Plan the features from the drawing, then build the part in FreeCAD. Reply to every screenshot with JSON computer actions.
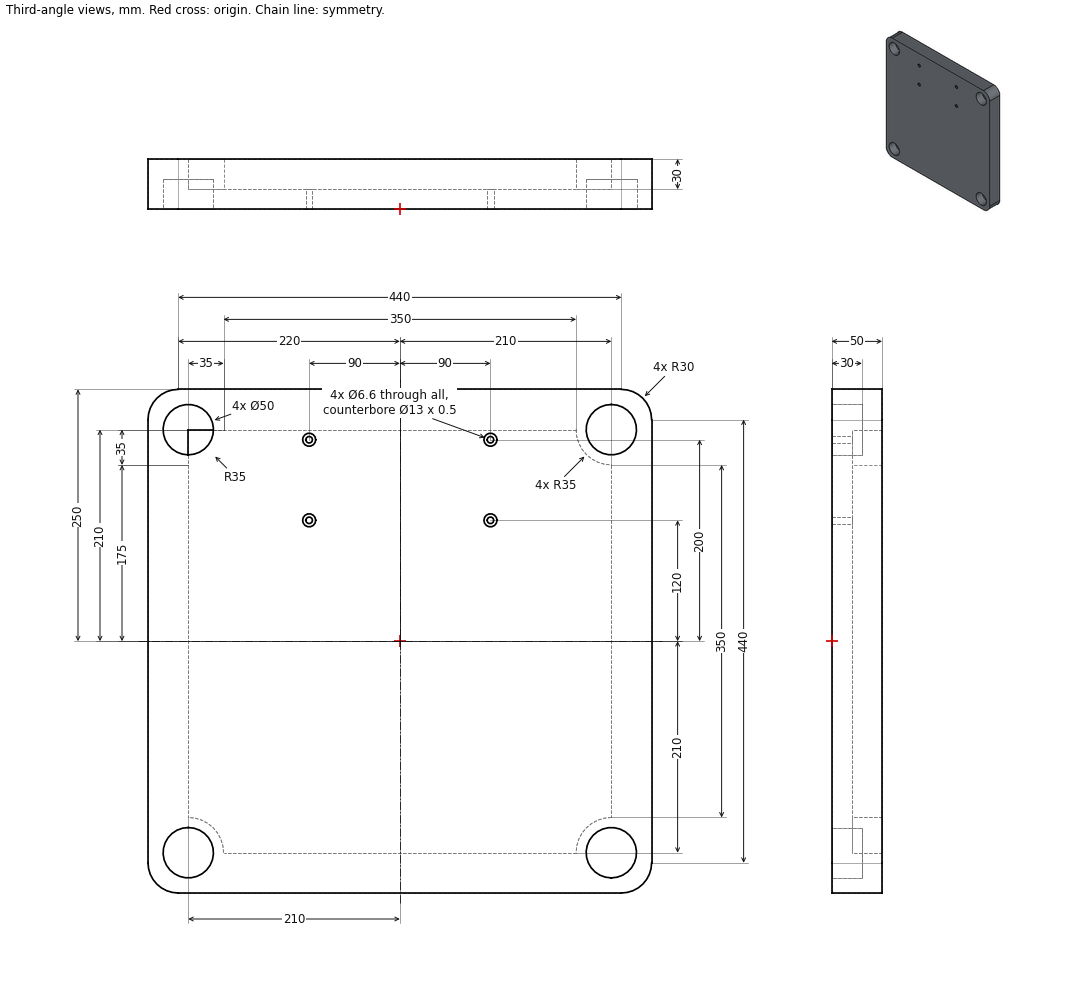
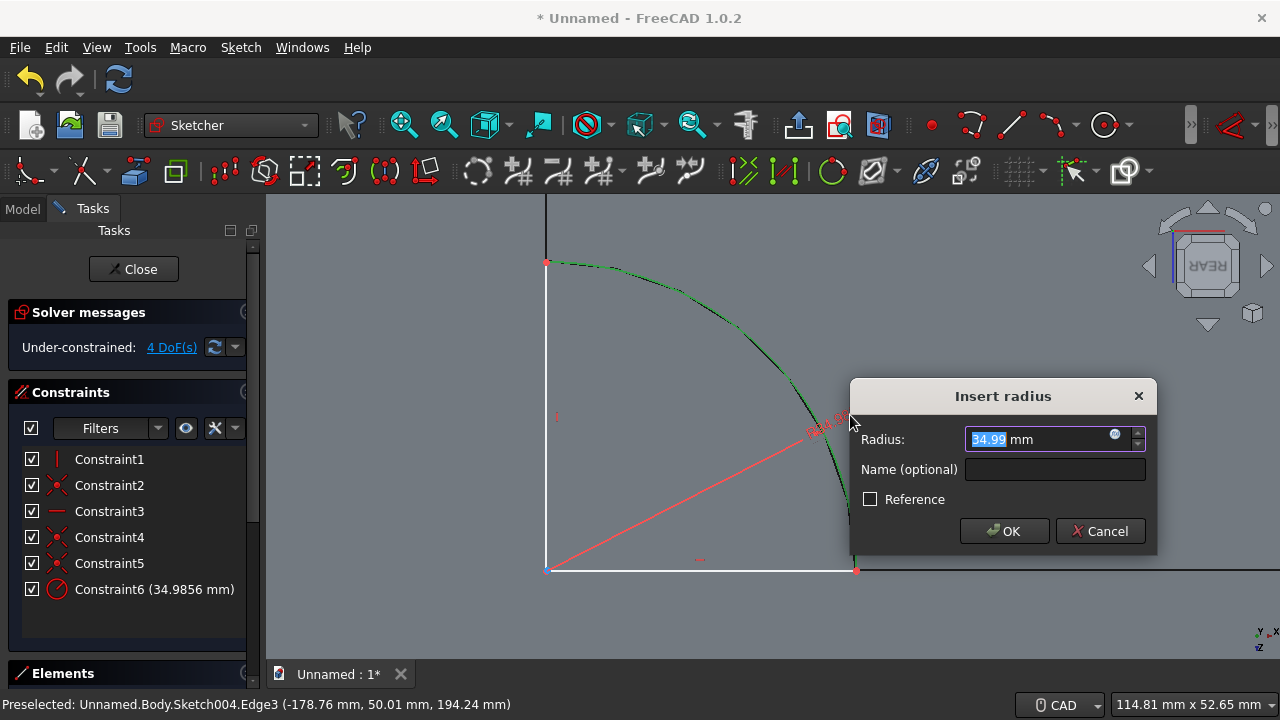
{"action": "type", "text": "35"}
{"action": "key", "text": "Return"}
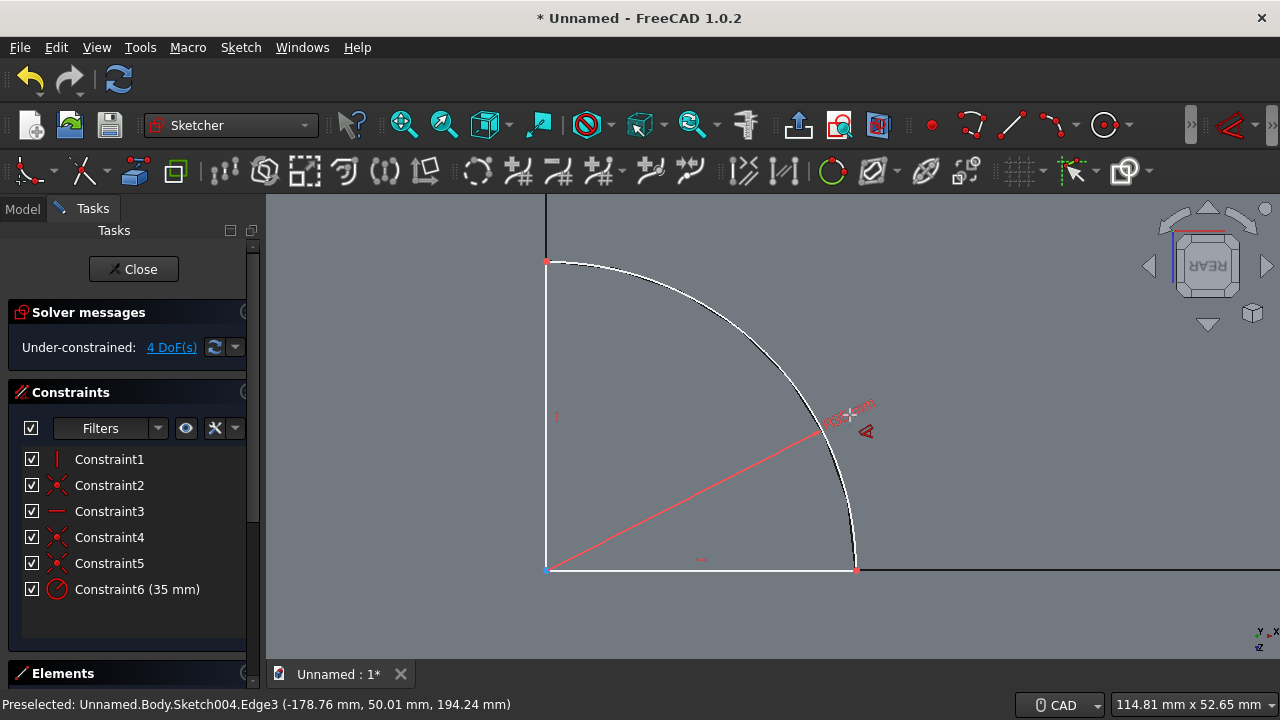
{"action": "left_click", "coordinate": [546, 355]}
{"action": "left_click", "coordinate": [512, 416]}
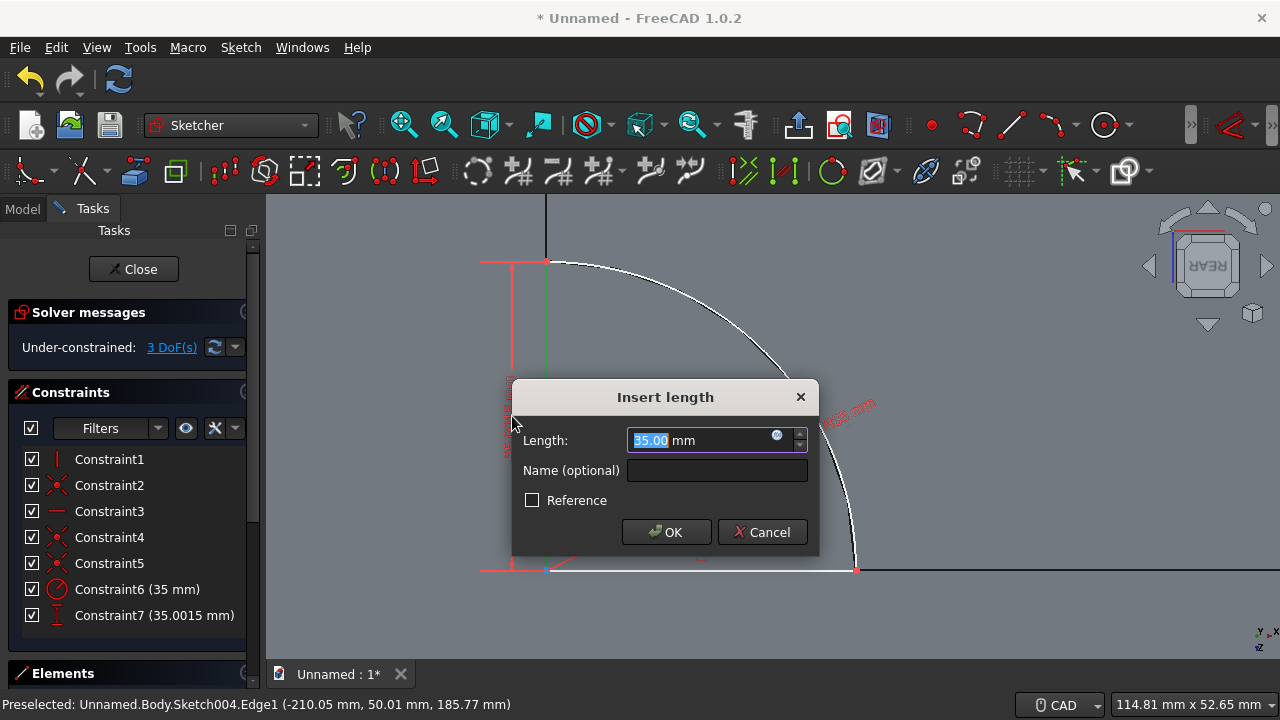
{"action": "type", "text": "35"}
{"action": "key", "text": "Return"}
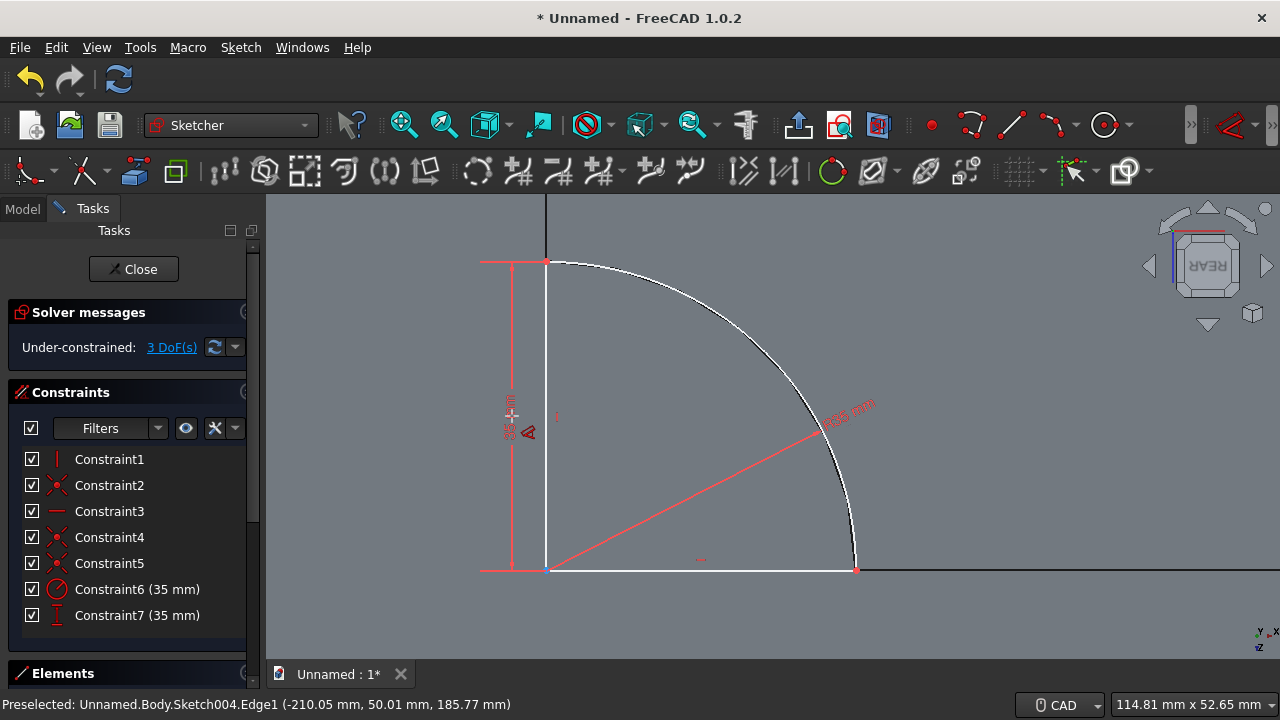
{"action": "left_click", "coordinate": [639, 571]}
{"action": "left_click", "coordinate": [701, 605]}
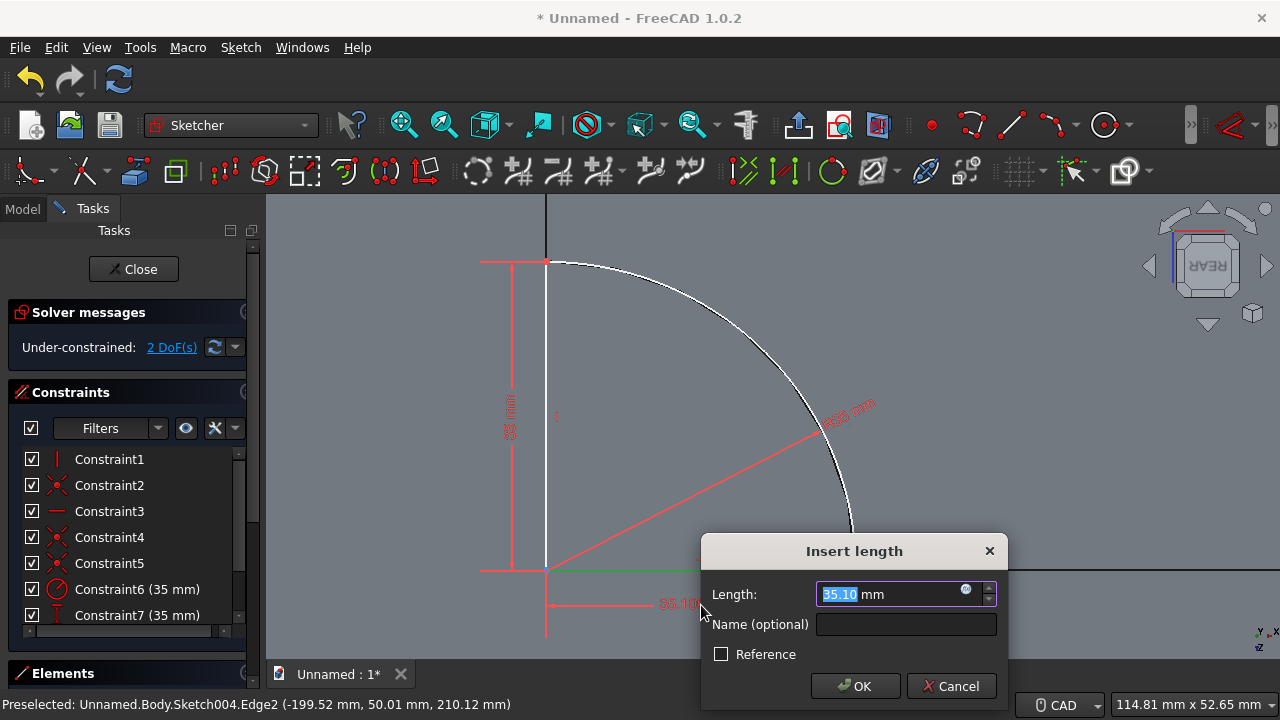
{"action": "type", "text": "35"}
{"action": "key", "text": "Return"}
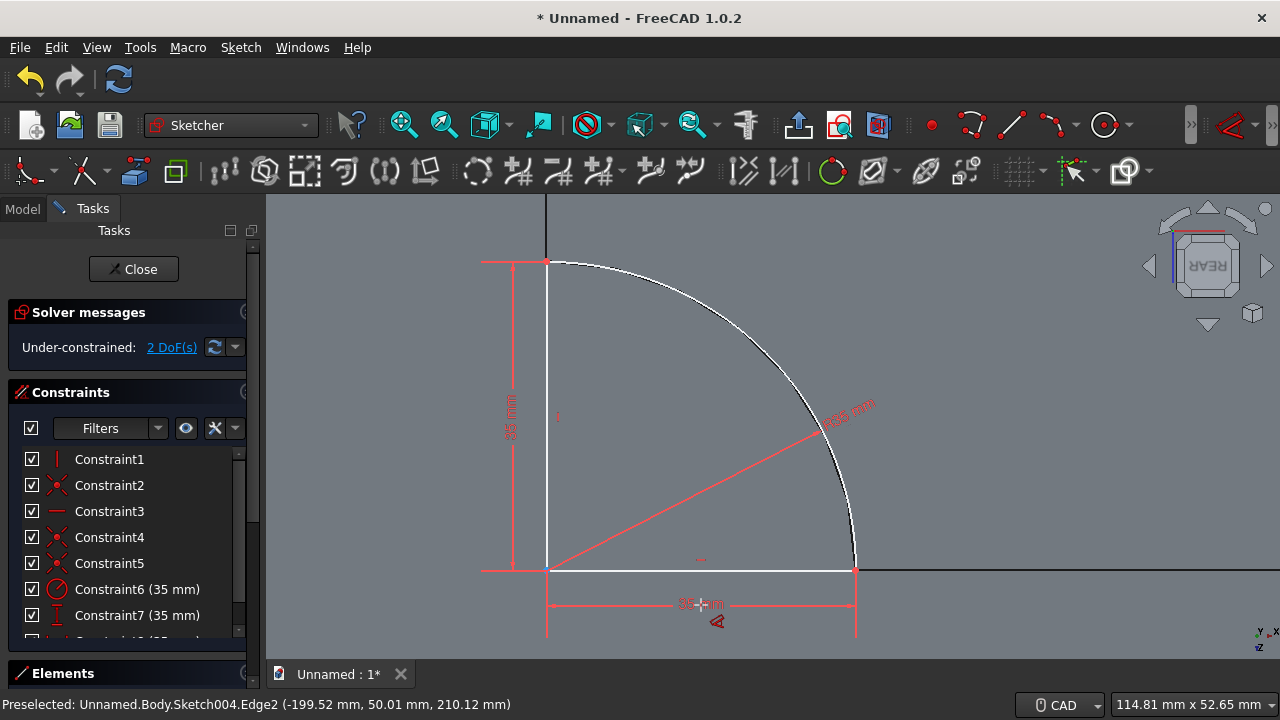
{"action": "left_click", "coordinate": [547, 262]}
{"action": "left_click", "coordinate": [831, 296]}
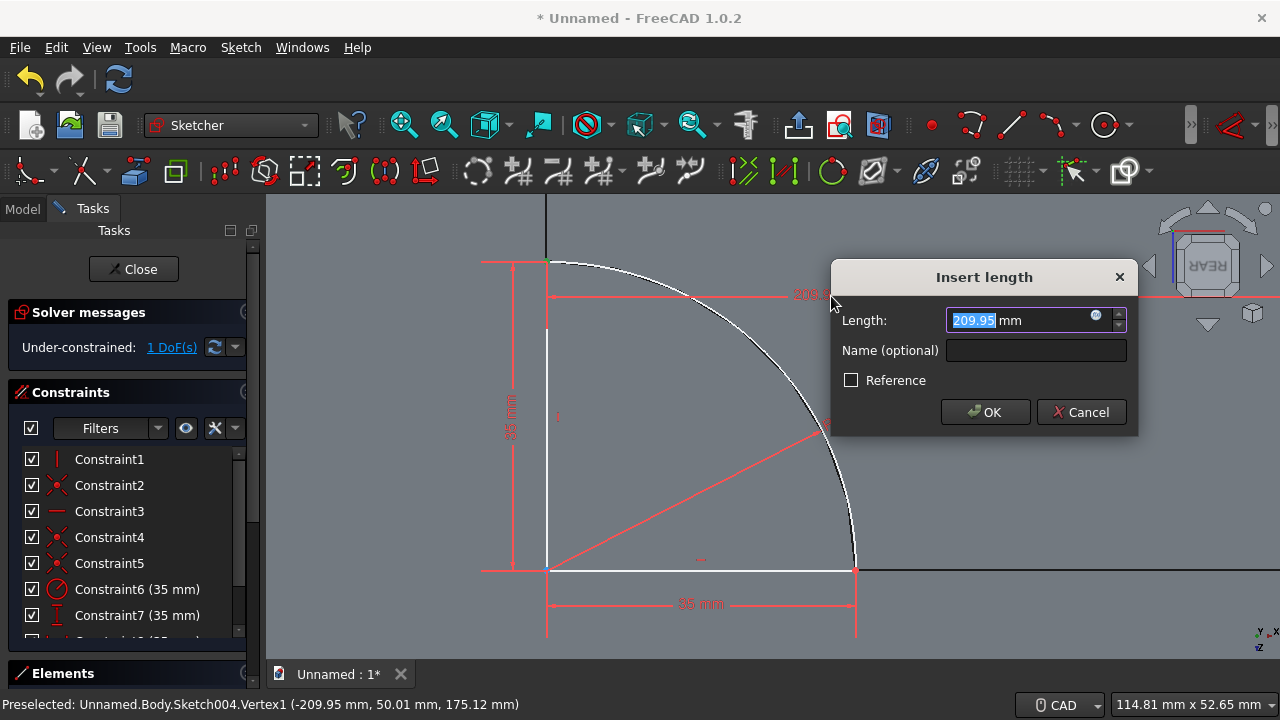
{"action": "type", "text": "210"}
{"action": "key", "text": "Return"}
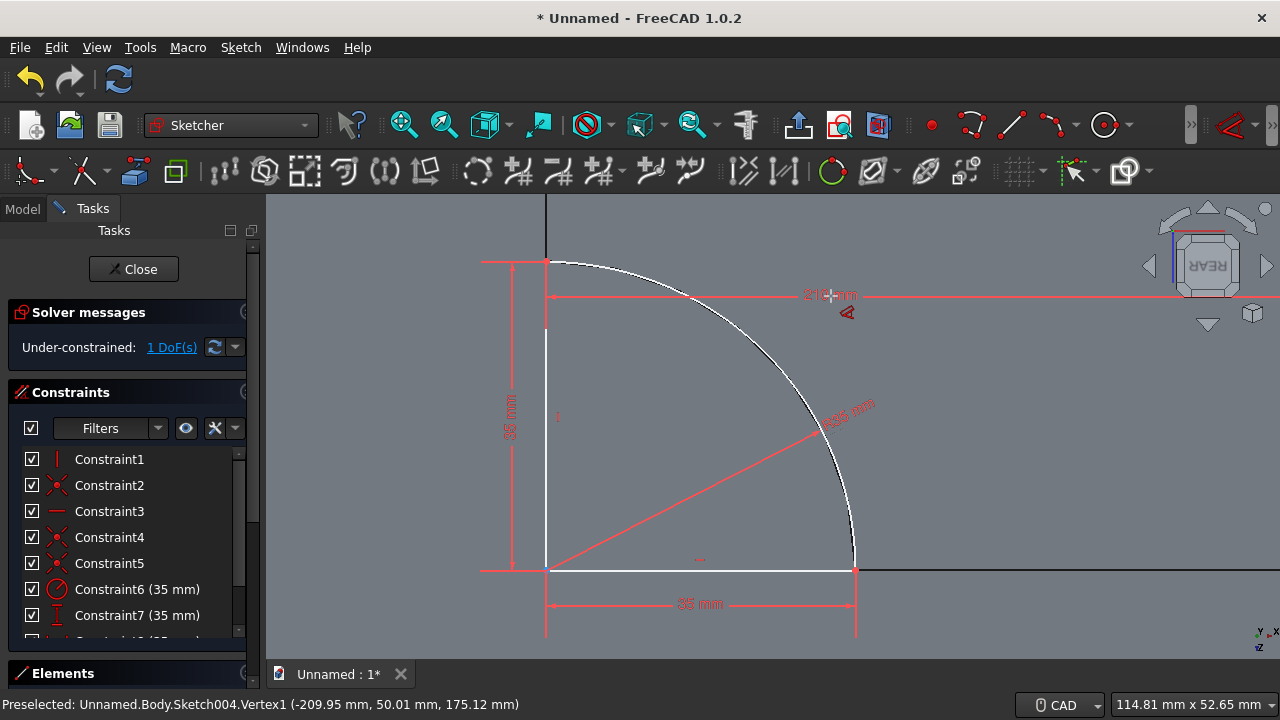
{"action": "left_click", "coordinate": [546, 262]}
{"action": "left_click", "coordinate": [512, 242]}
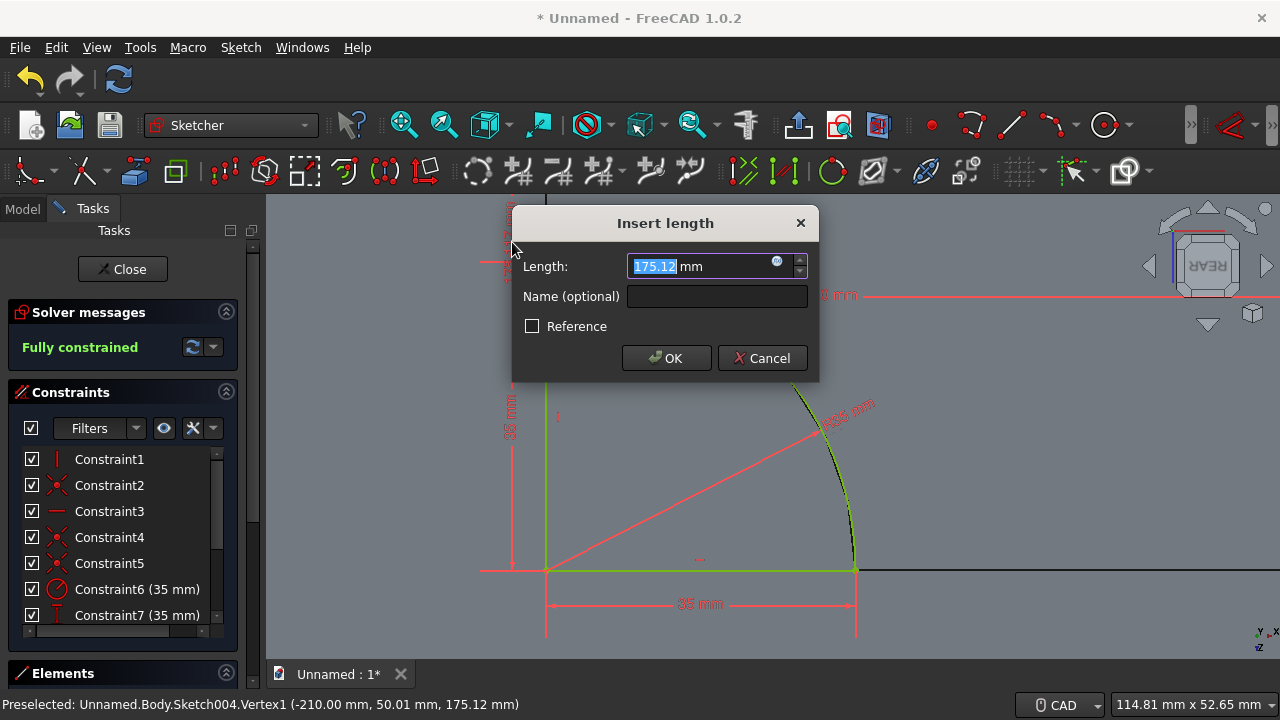
{"action": "type", "text": "175"}
{"action": "key", "text": "Return"}
{"action": "key", "text": "Escape"}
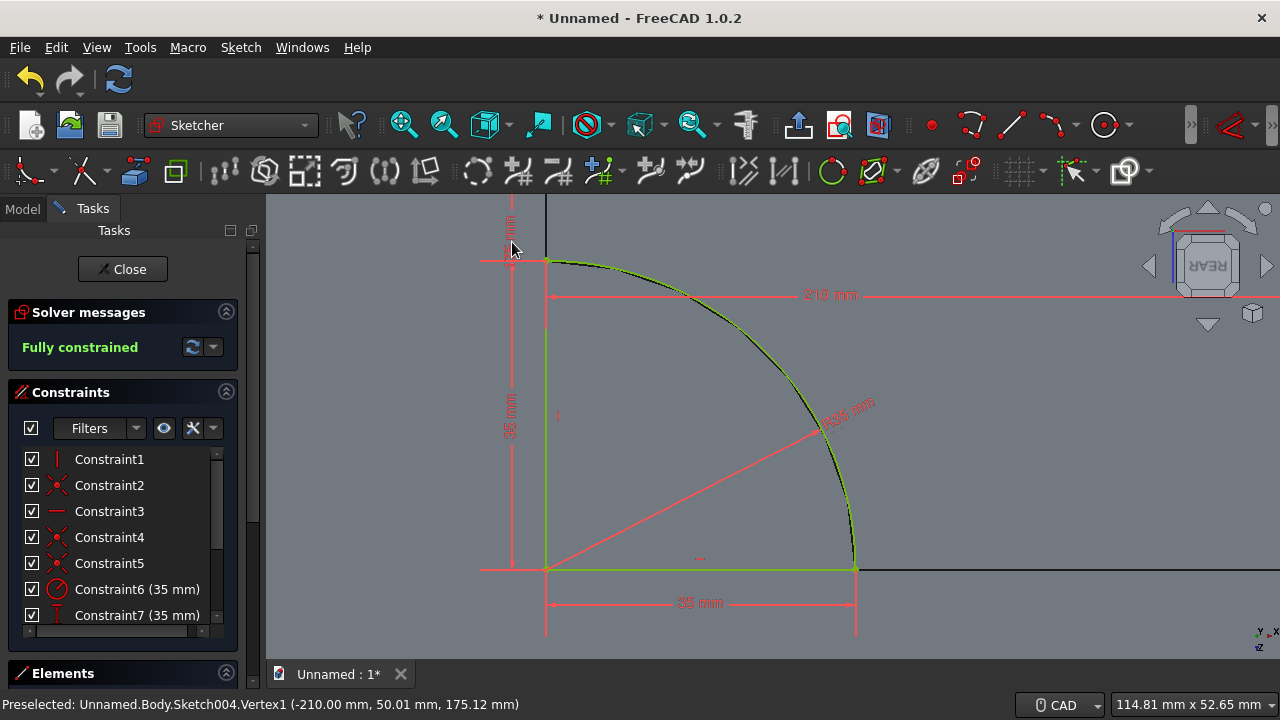
{"action": "left_click", "coordinate": [123, 269]}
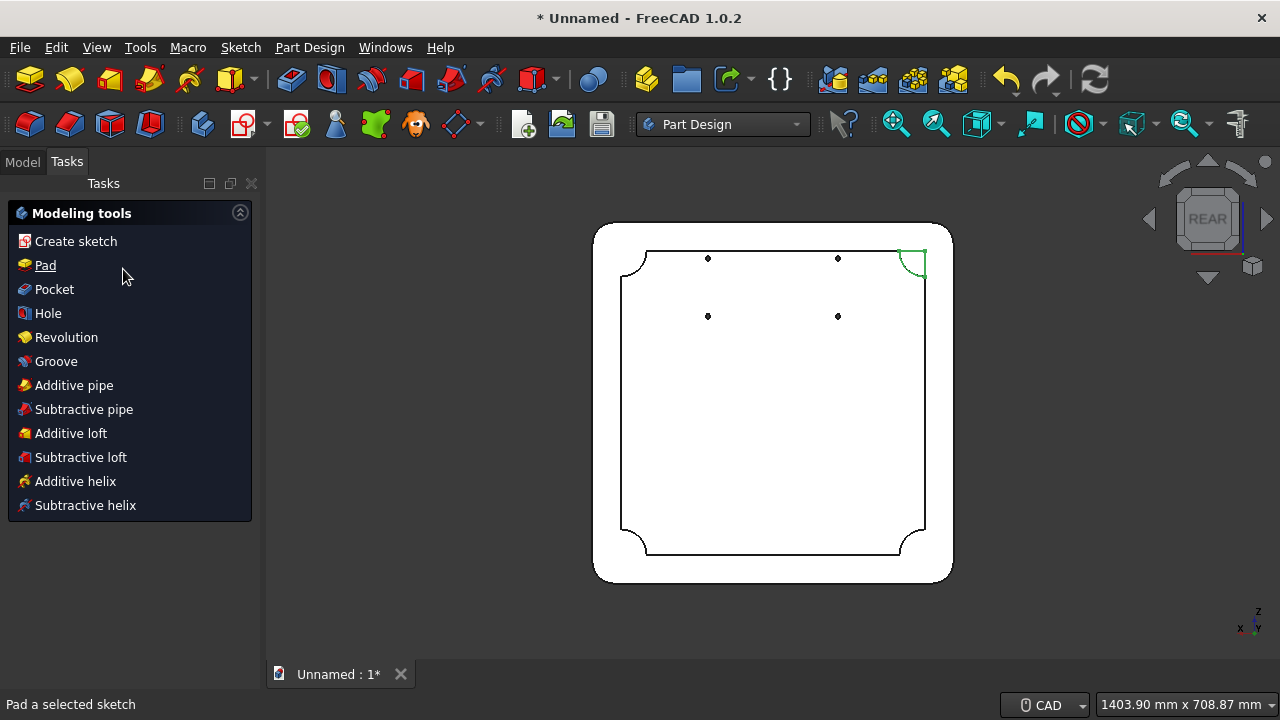
{"action": "left_click", "coordinate": [292, 80]}